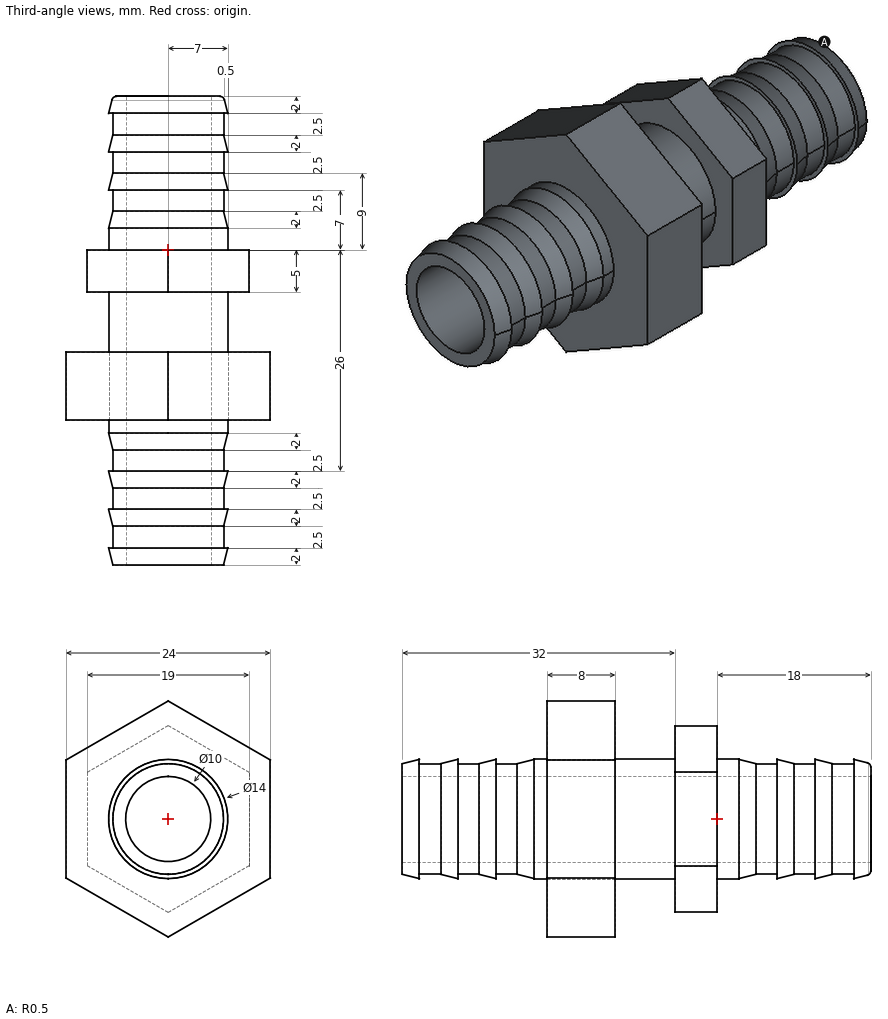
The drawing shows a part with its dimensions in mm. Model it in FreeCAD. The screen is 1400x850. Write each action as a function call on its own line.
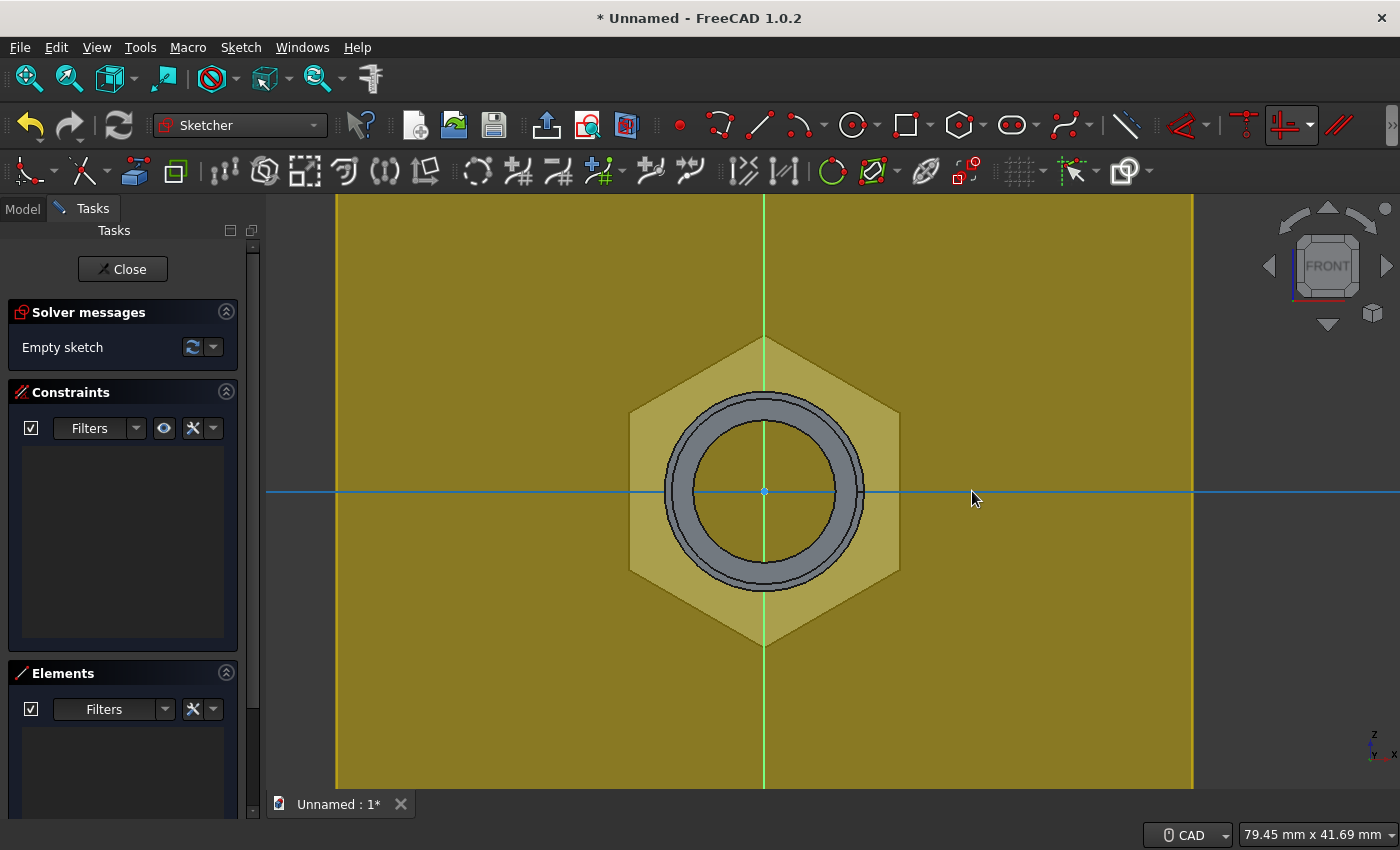
click(960, 126)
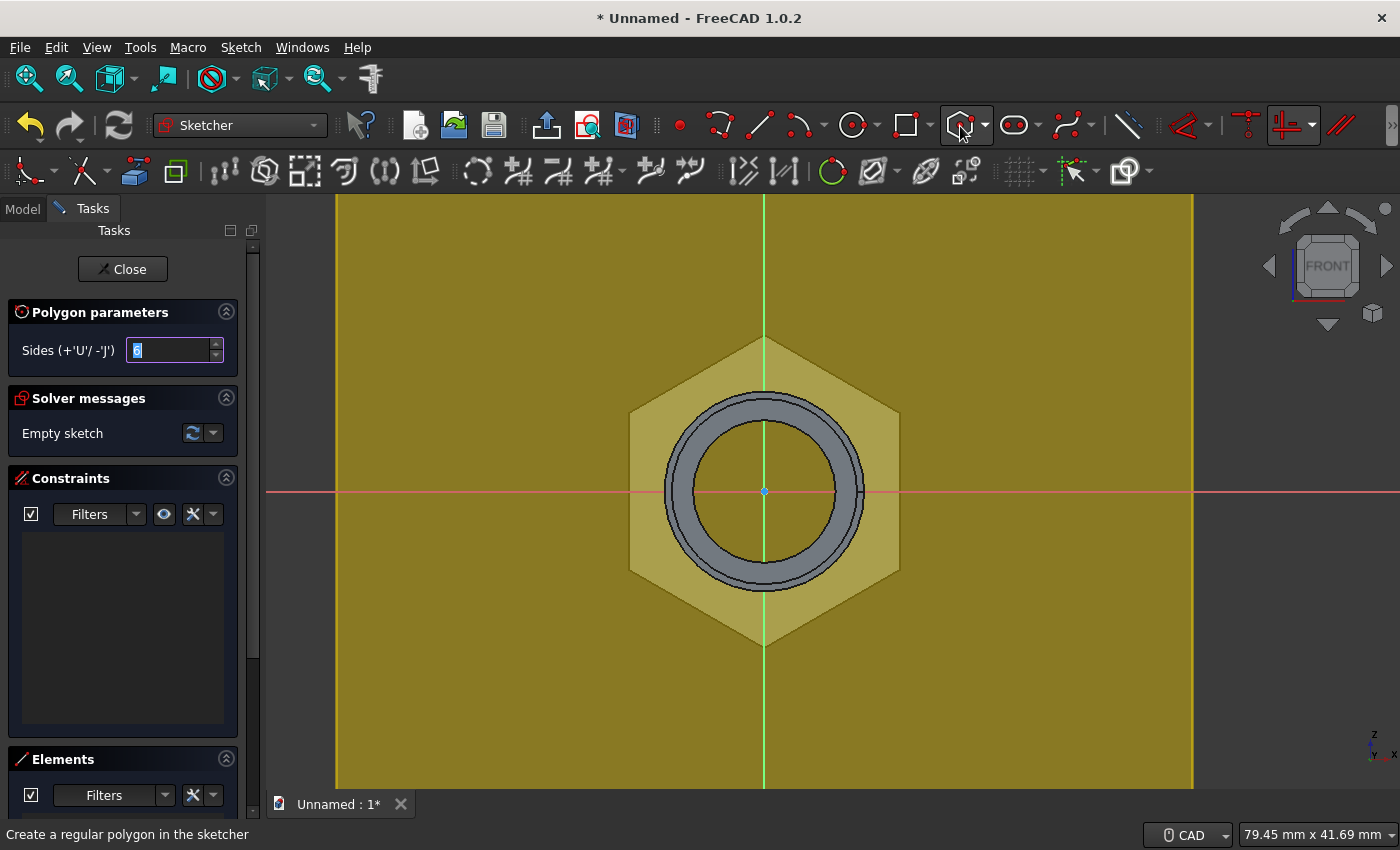
click(764, 491)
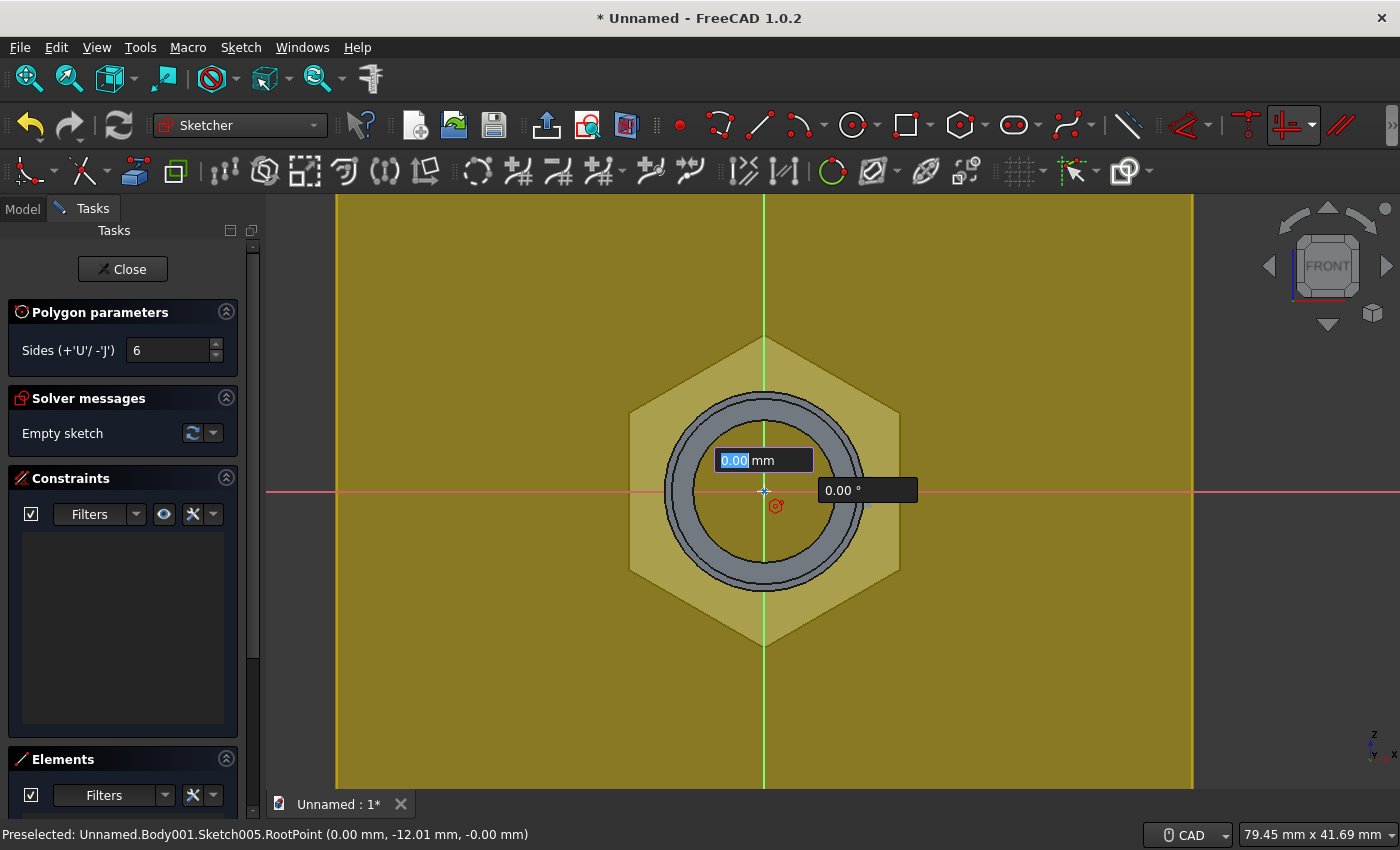
click(764, 689)
right_click(764, 689)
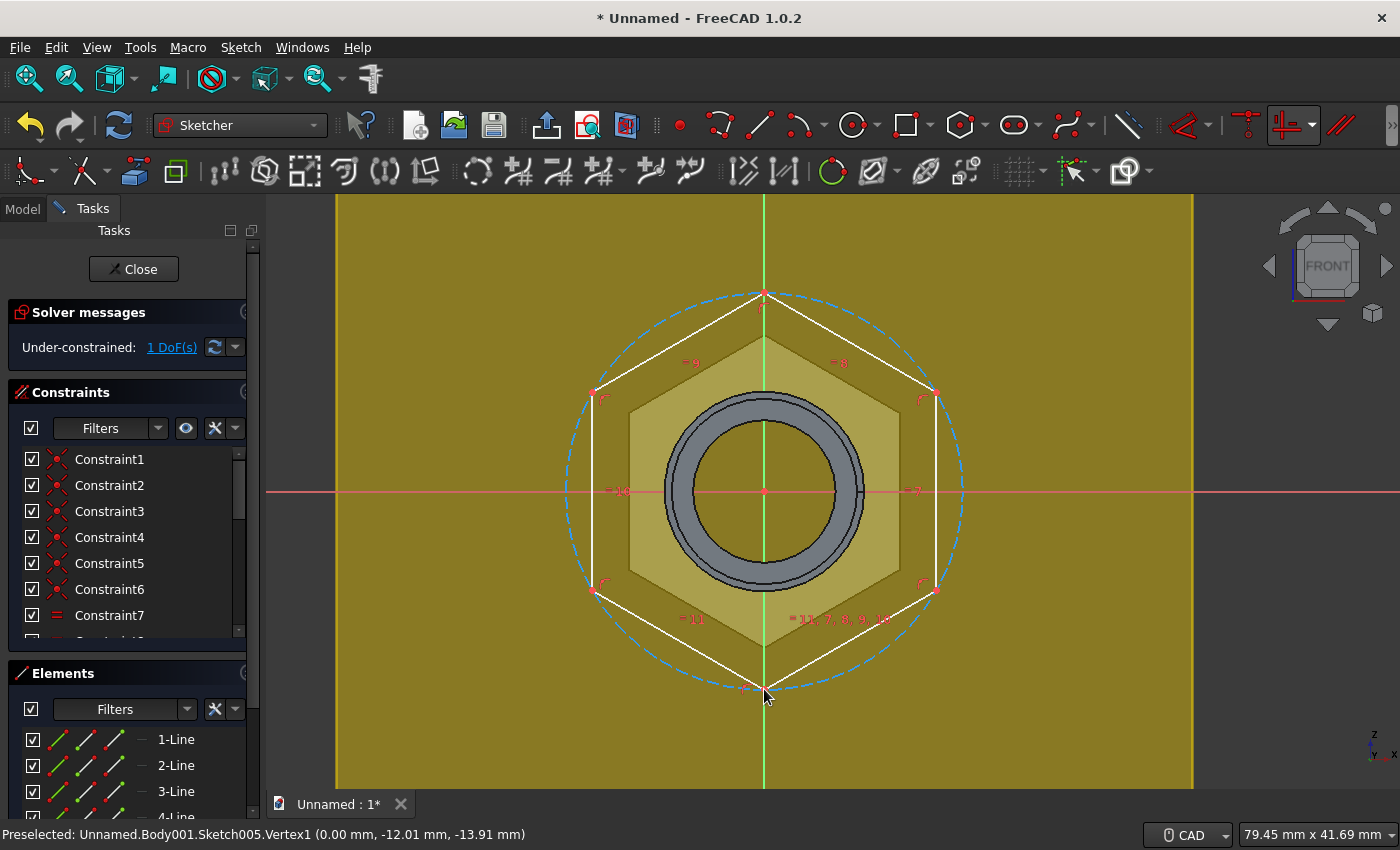
click(854, 126)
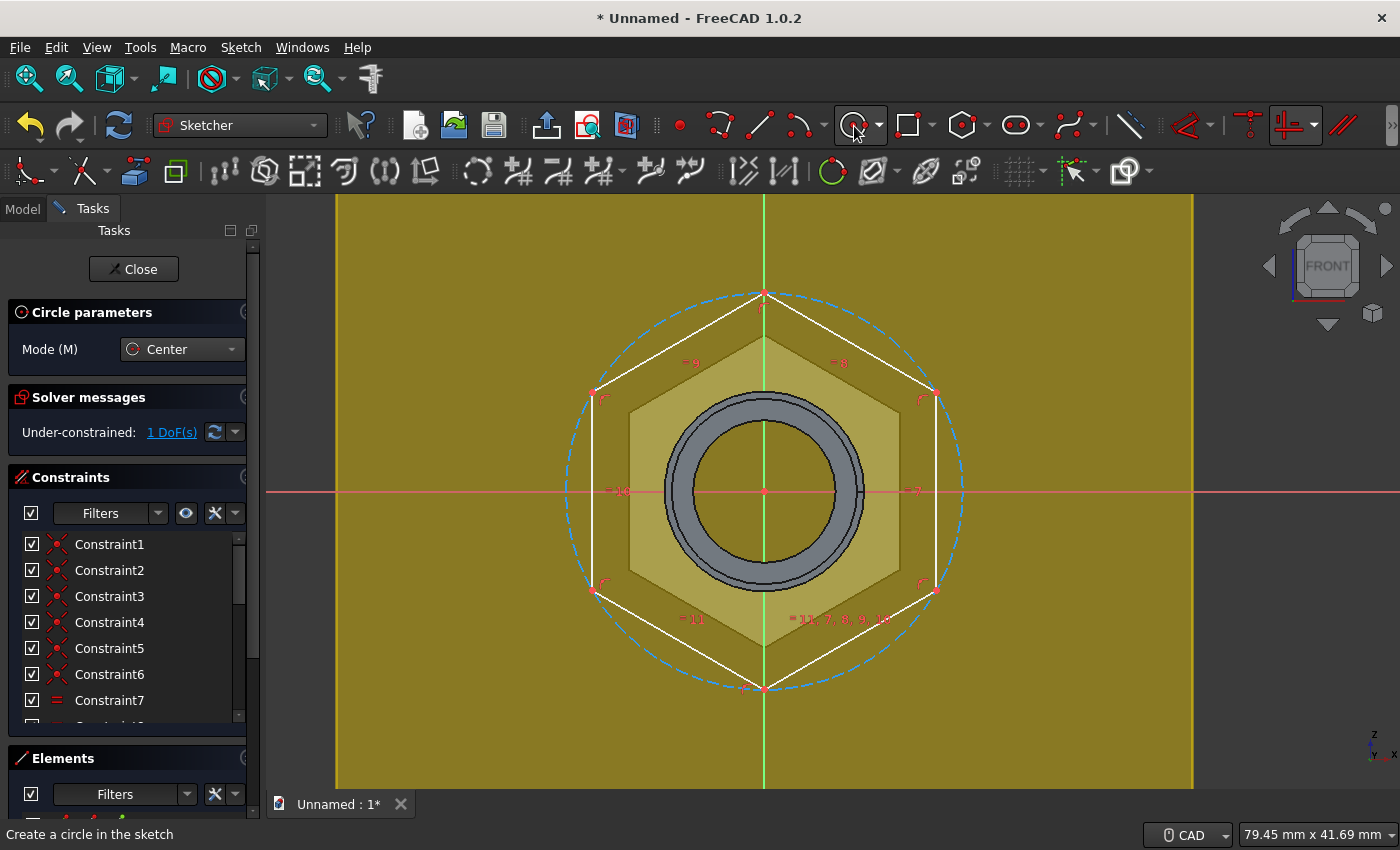
click(764, 491)
move(835, 421)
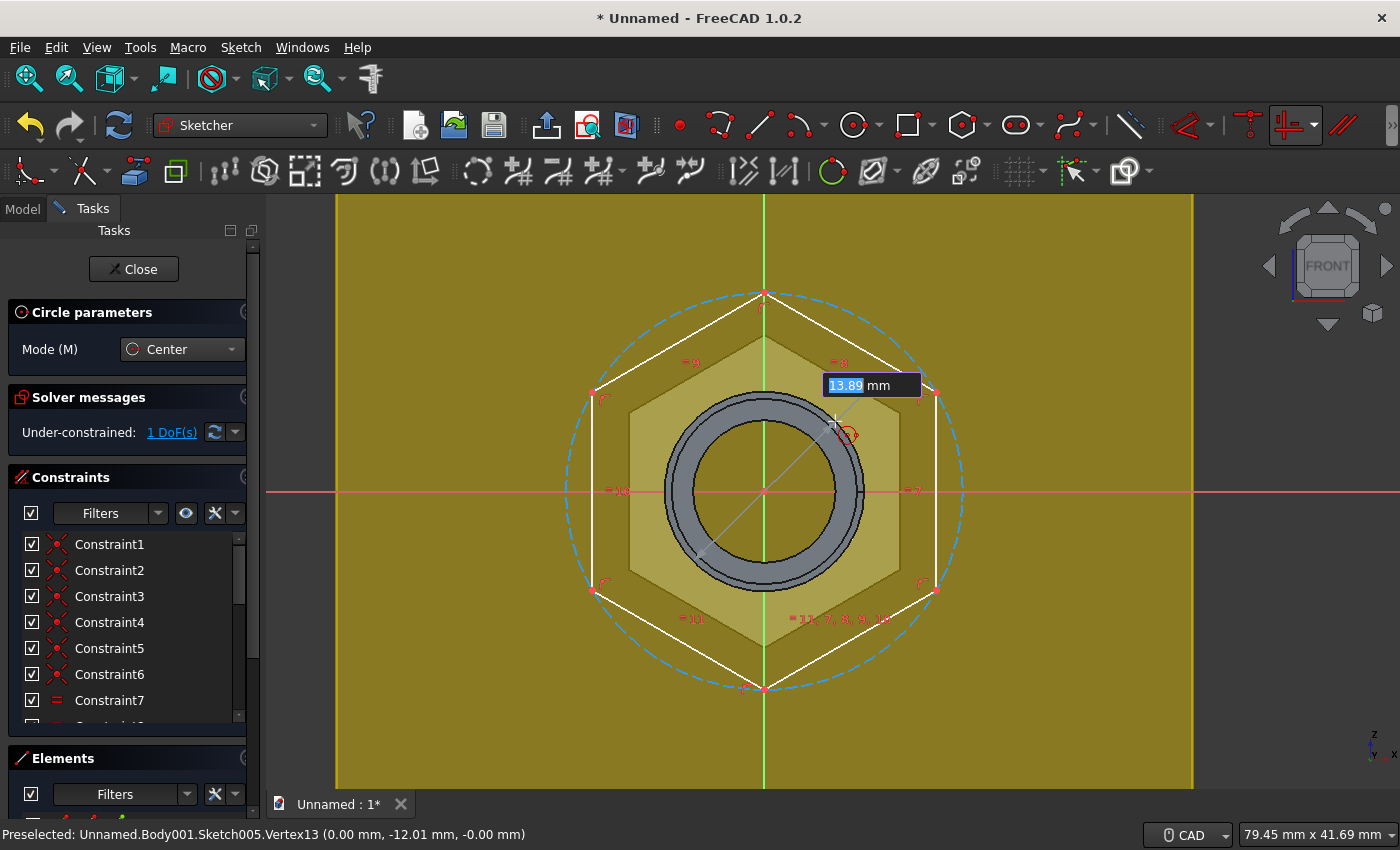
text(14)
key(Return)
key(Escape)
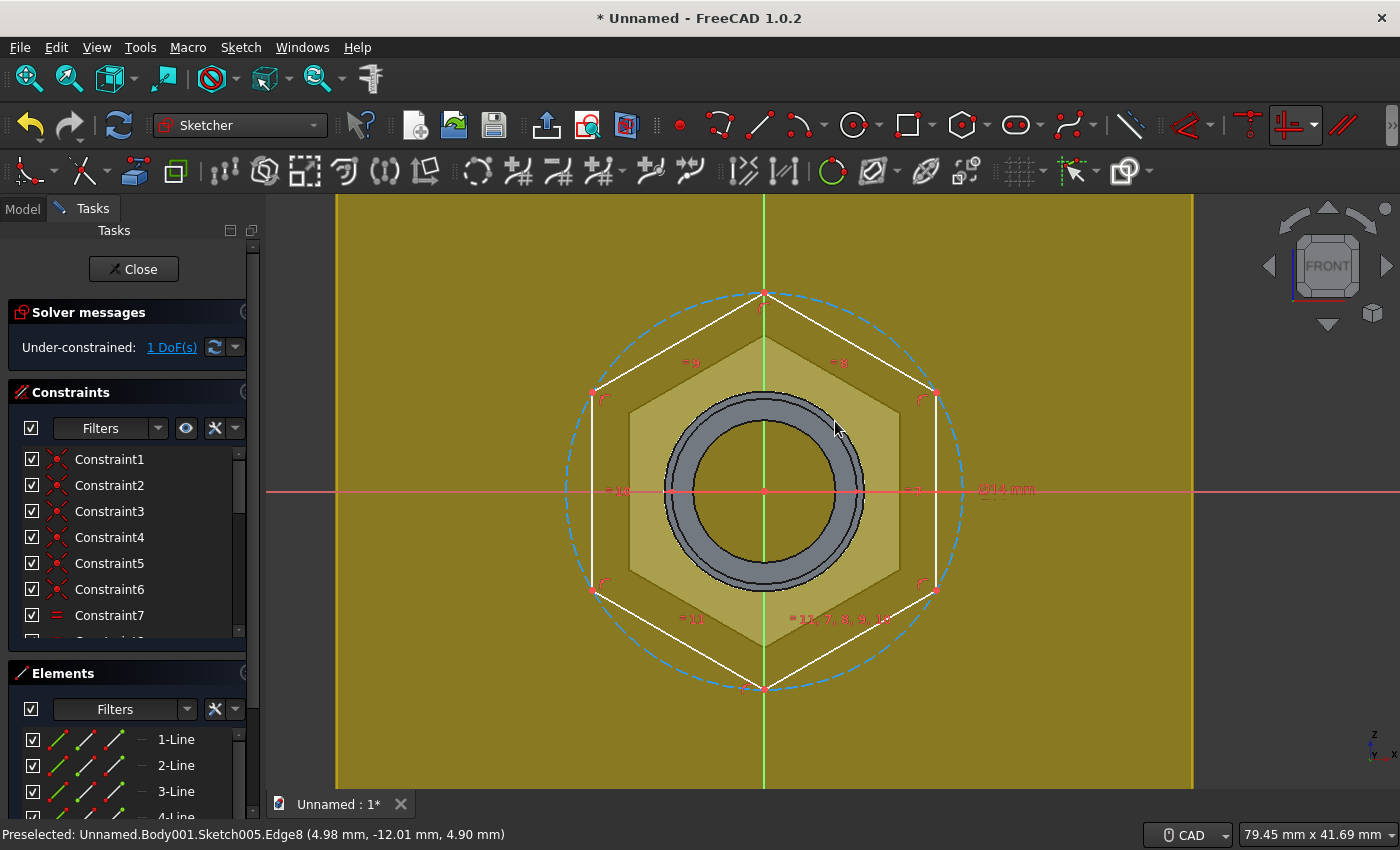
click(1186, 126)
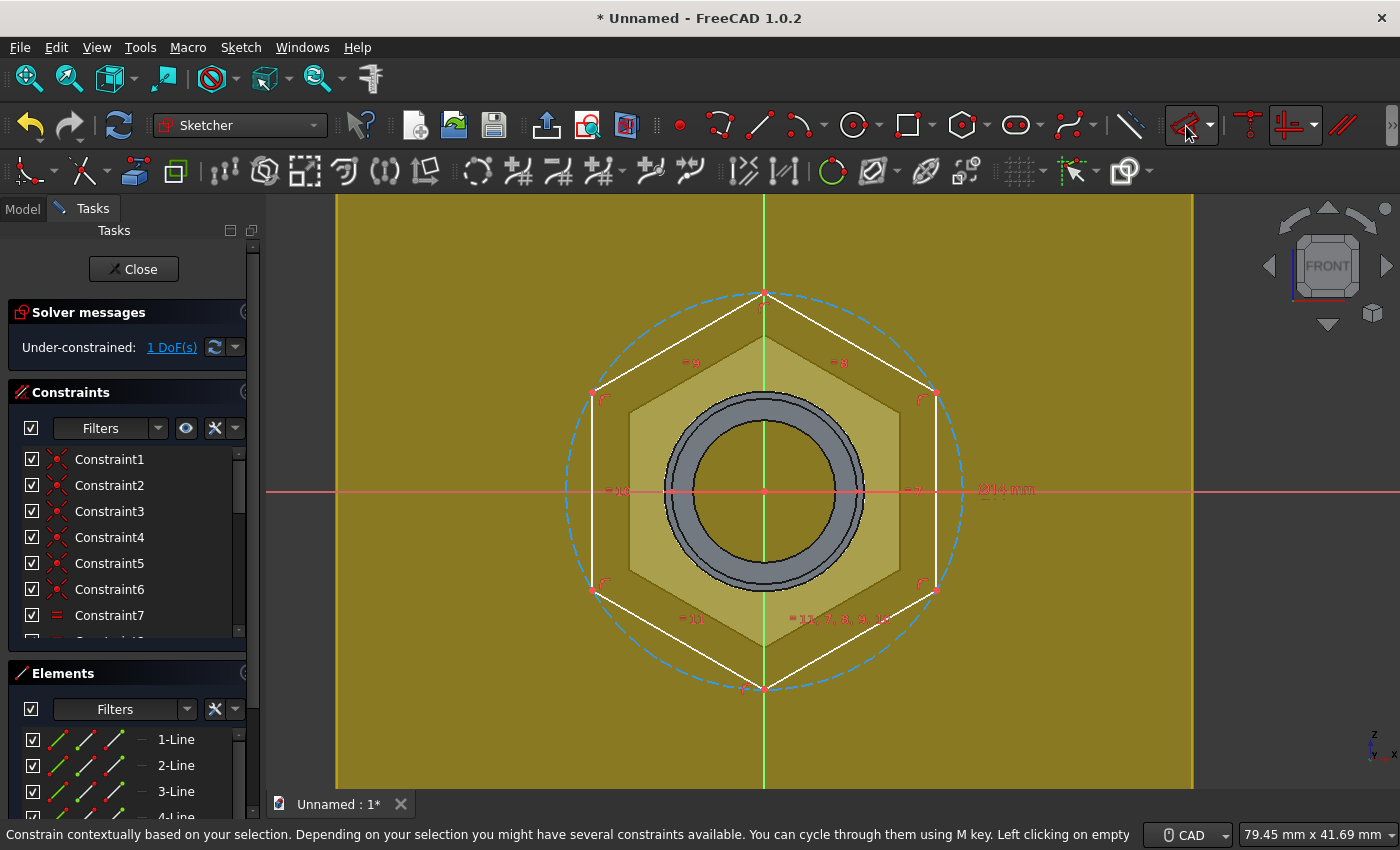
click(592, 392)